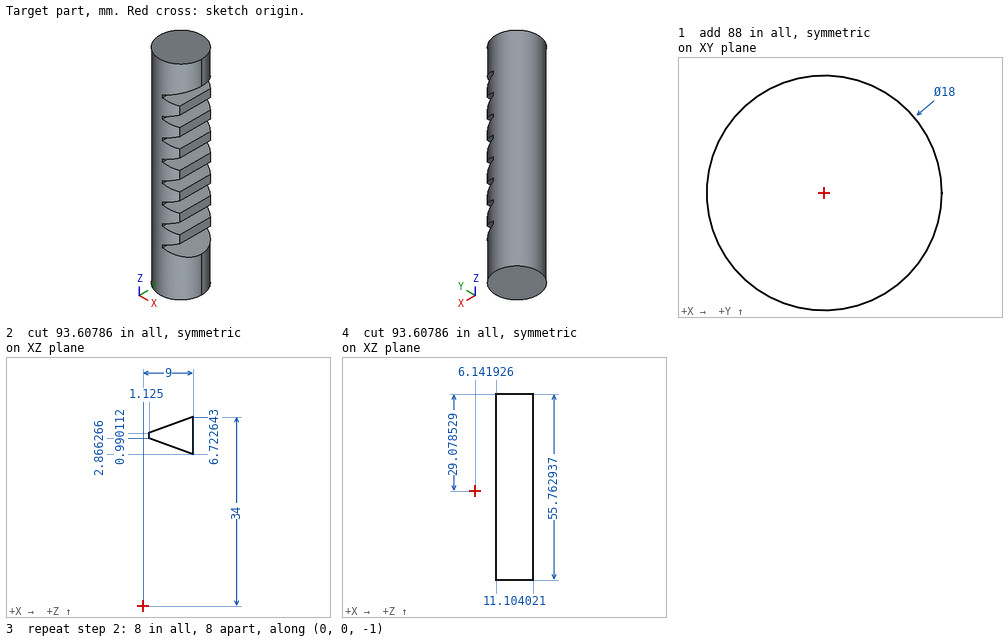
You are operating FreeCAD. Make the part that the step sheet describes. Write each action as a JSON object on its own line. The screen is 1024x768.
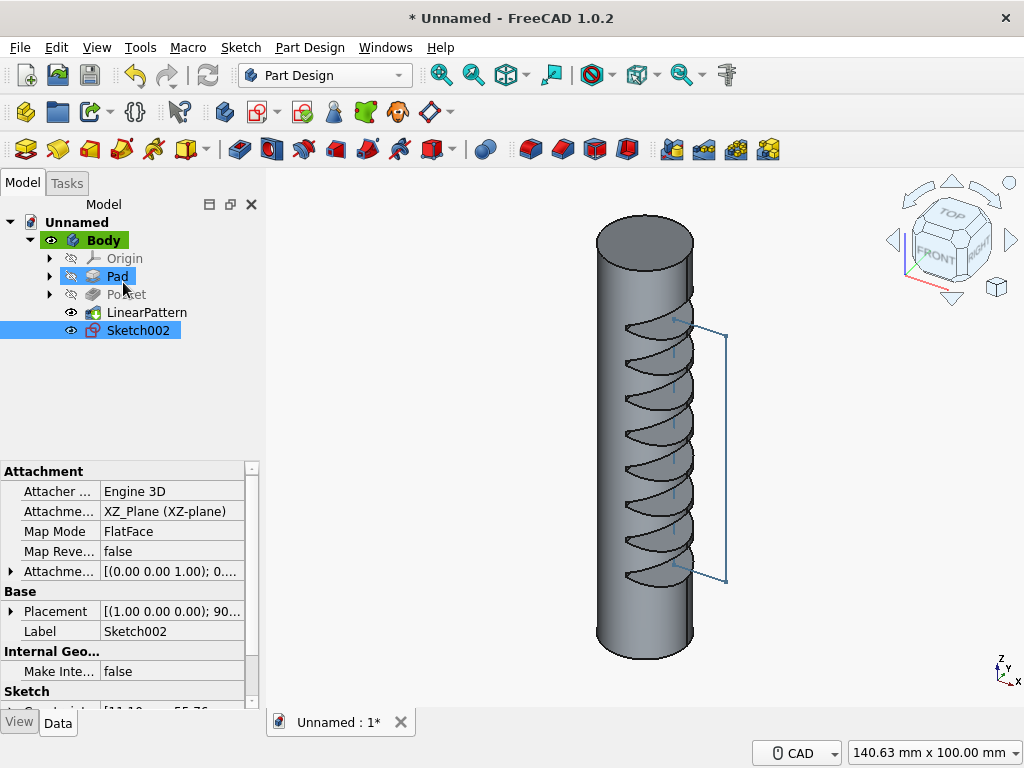
{"action": "left_click", "coordinate": [240, 150]}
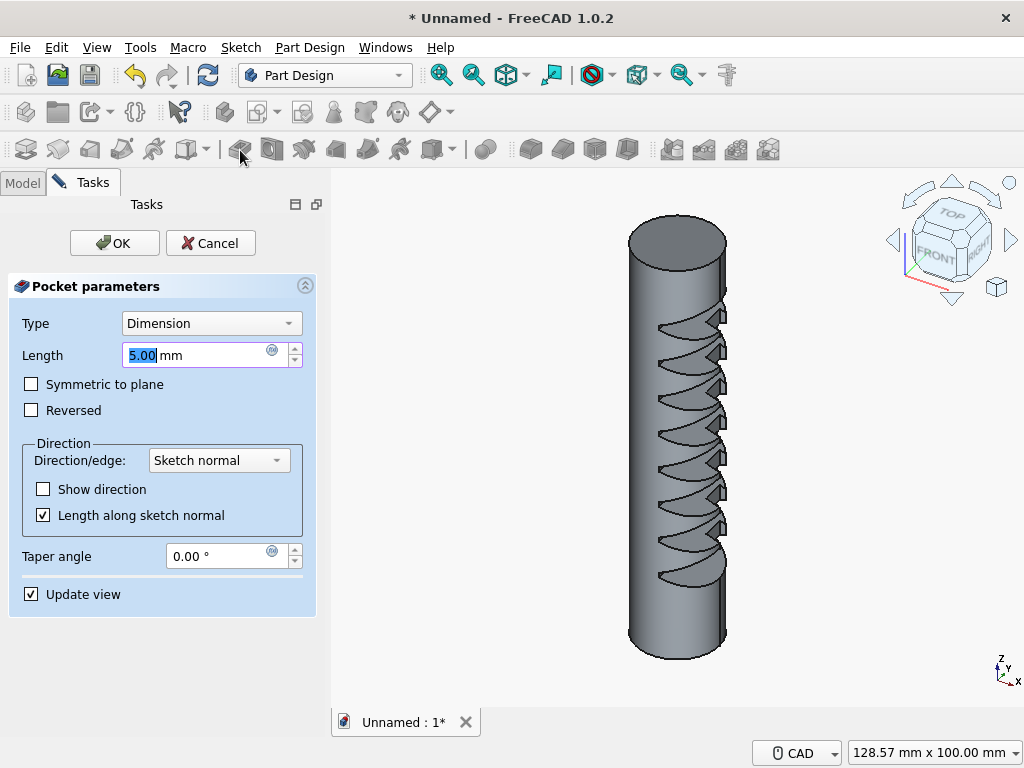
{"action": "type", "text": "93.60786"}
{"action": "key", "text": "Tab"}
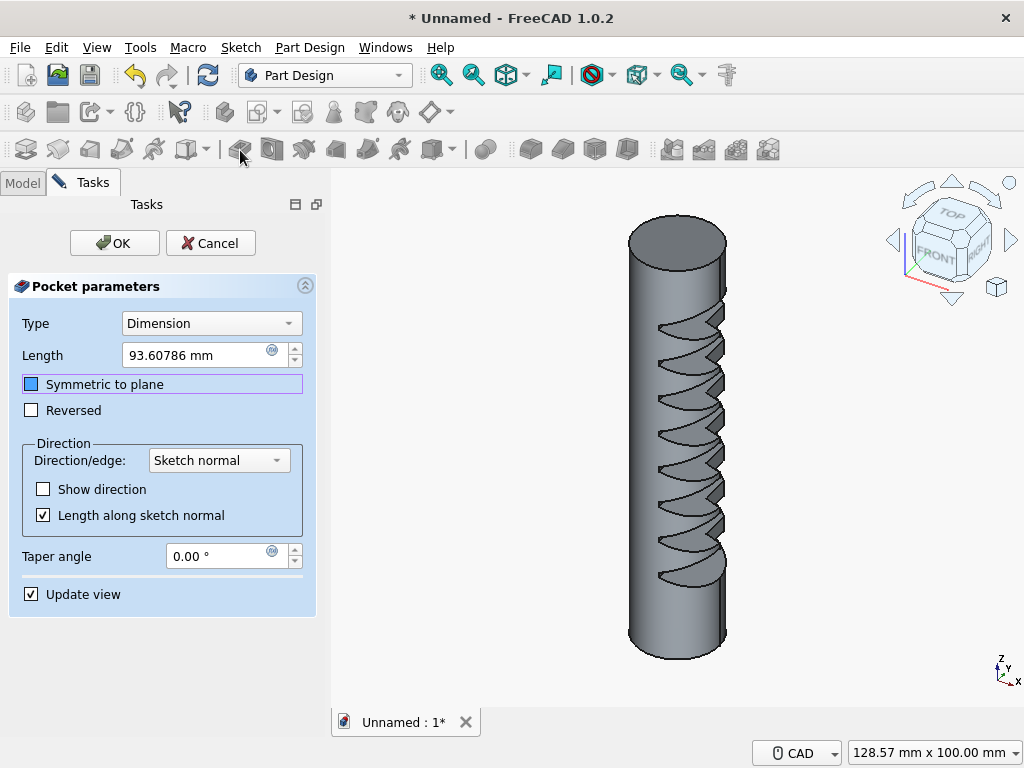
{"action": "left_click", "coordinate": [30, 384]}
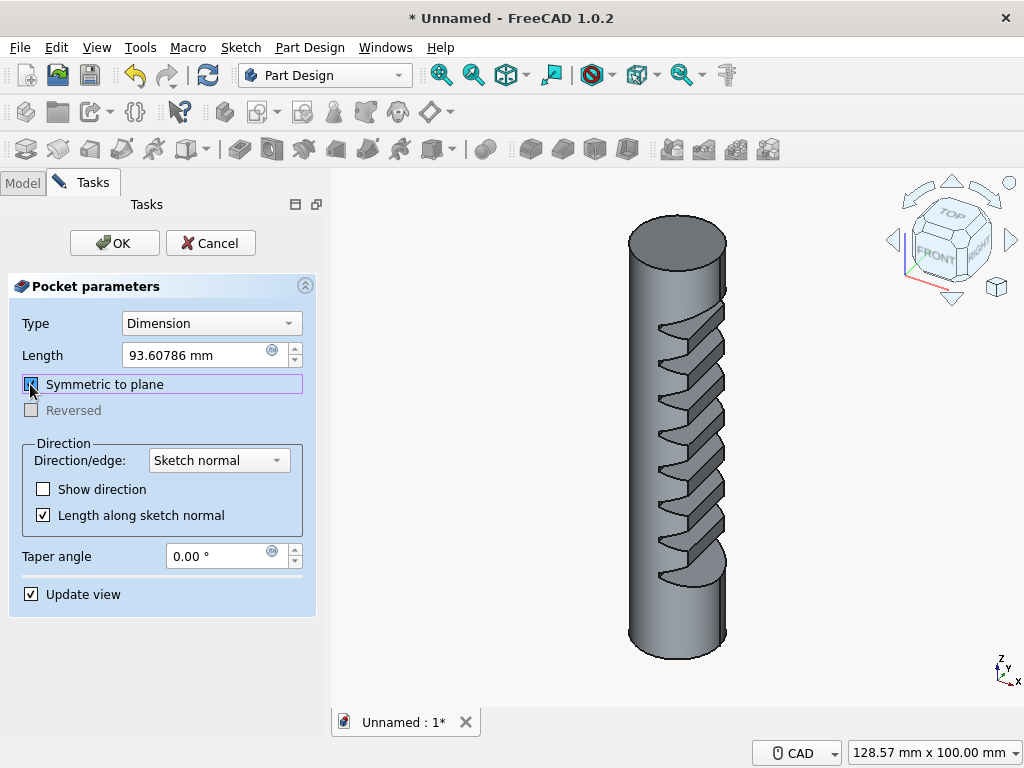
{"action": "left_click", "coordinate": [115, 243]}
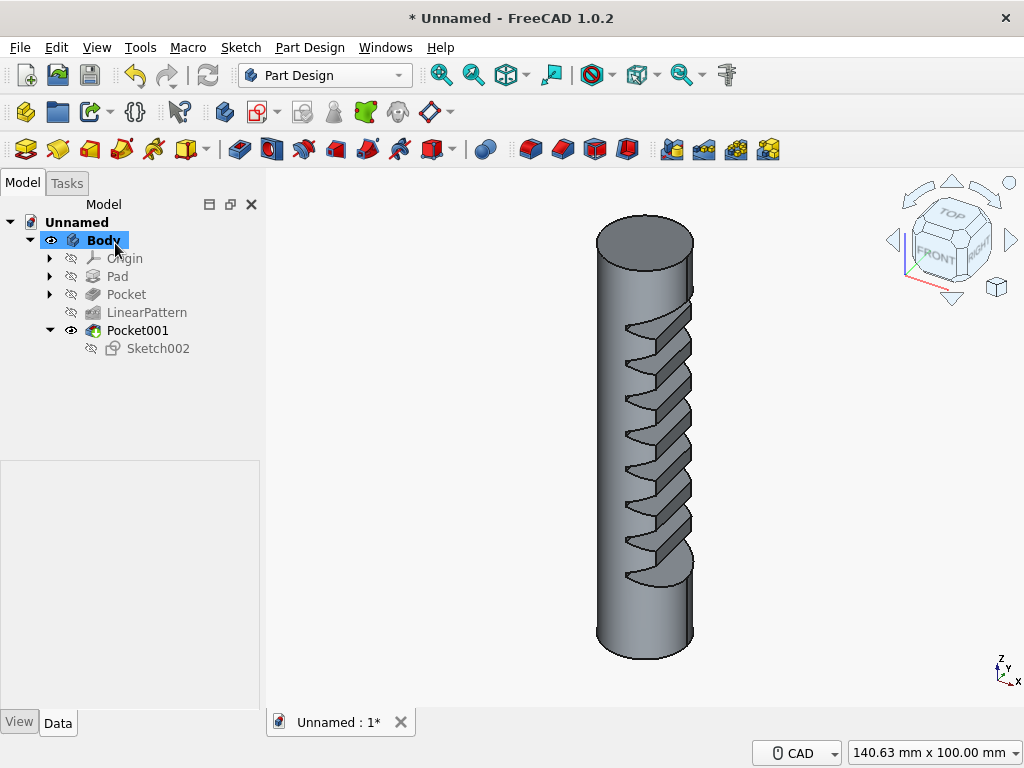
{"action": "key", "text": "0"}